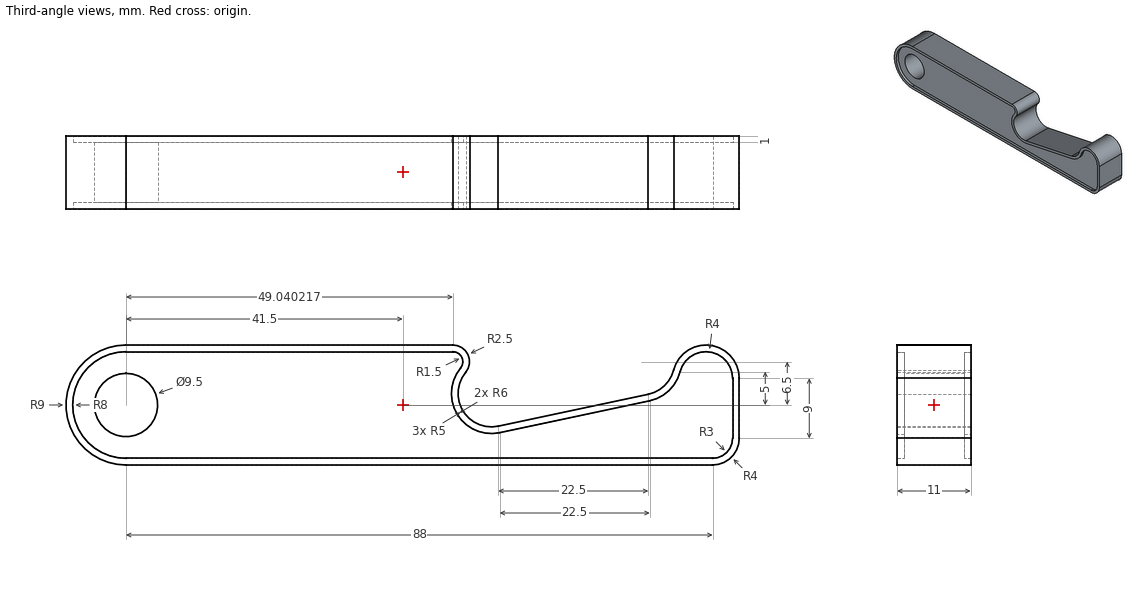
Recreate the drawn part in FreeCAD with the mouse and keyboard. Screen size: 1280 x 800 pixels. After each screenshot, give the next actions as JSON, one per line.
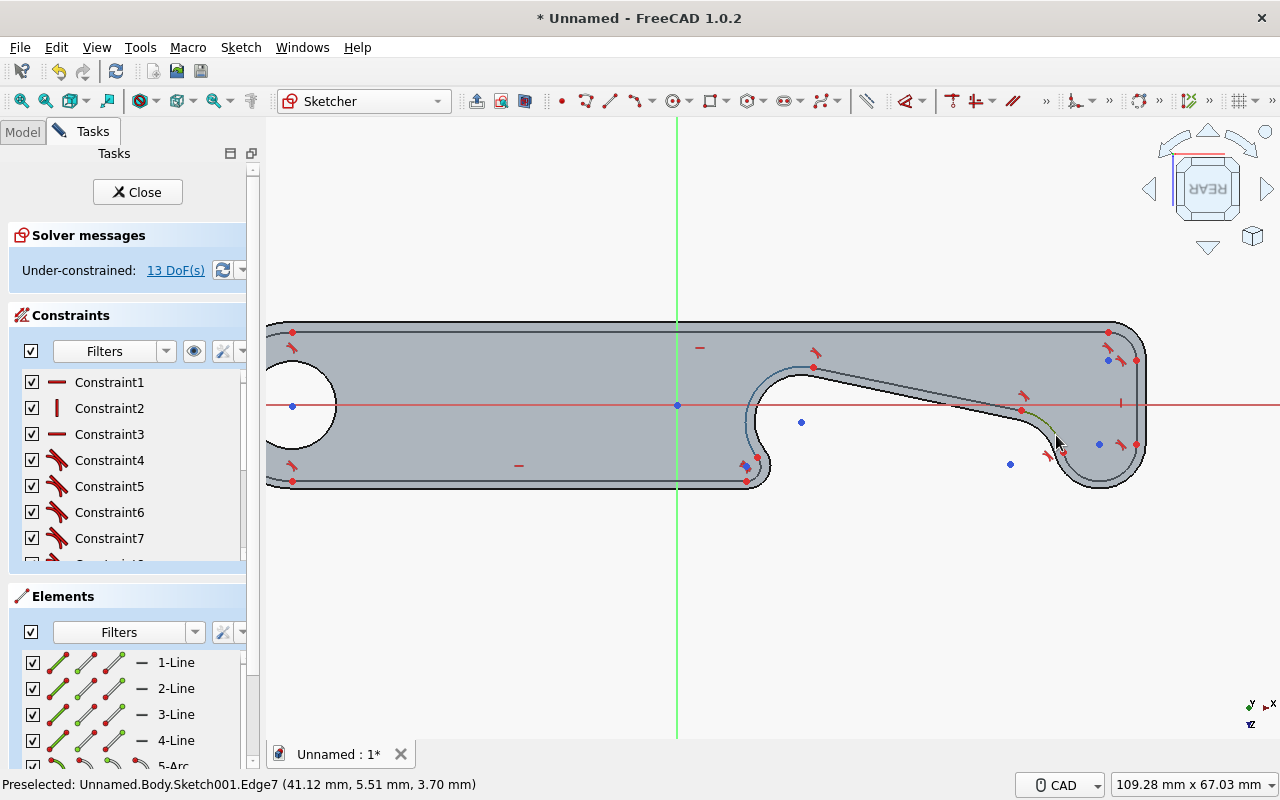
{"action": "key", "text": "e"}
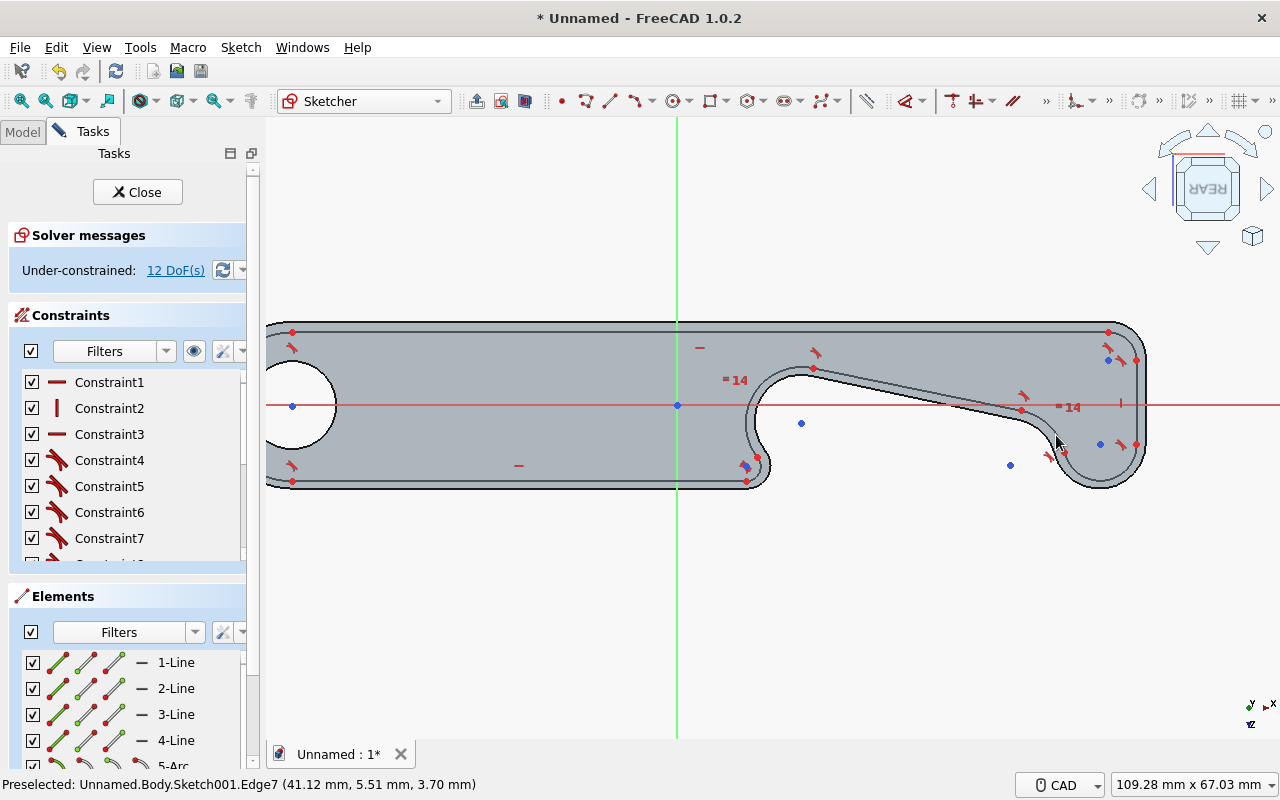
{"action": "scroll", "coordinate": [760, 474], "scroll_direction": "down", "scroll_amount": 2}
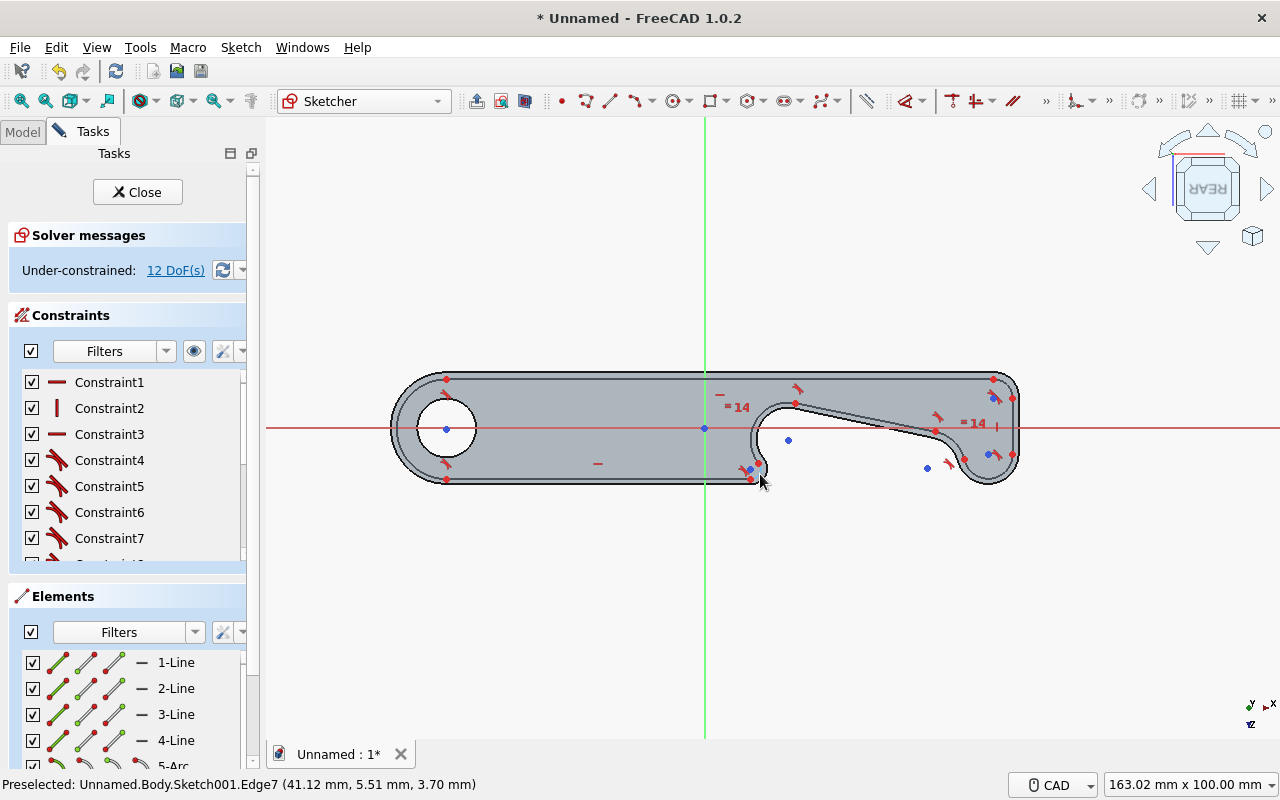
{"action": "left_click", "coordinate": [447, 429]}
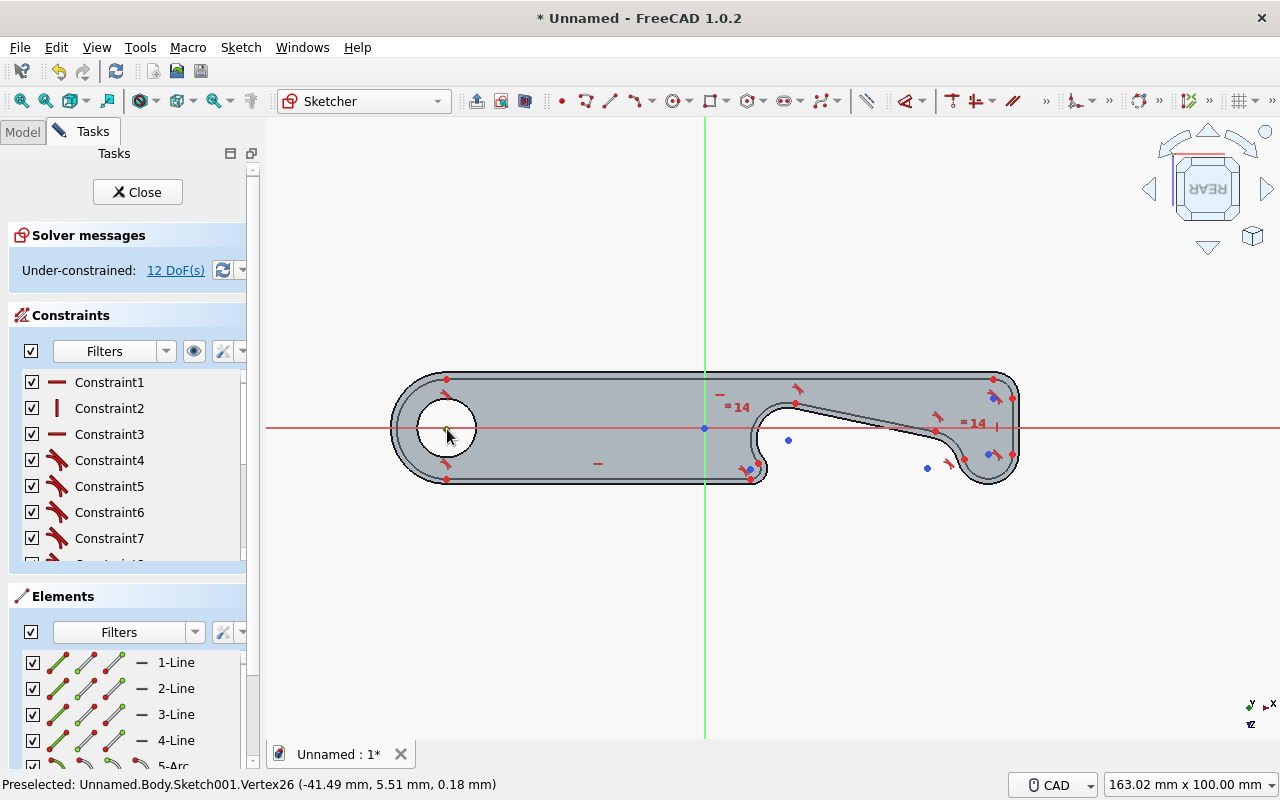
{"action": "left_click", "coordinate": [353, 428]}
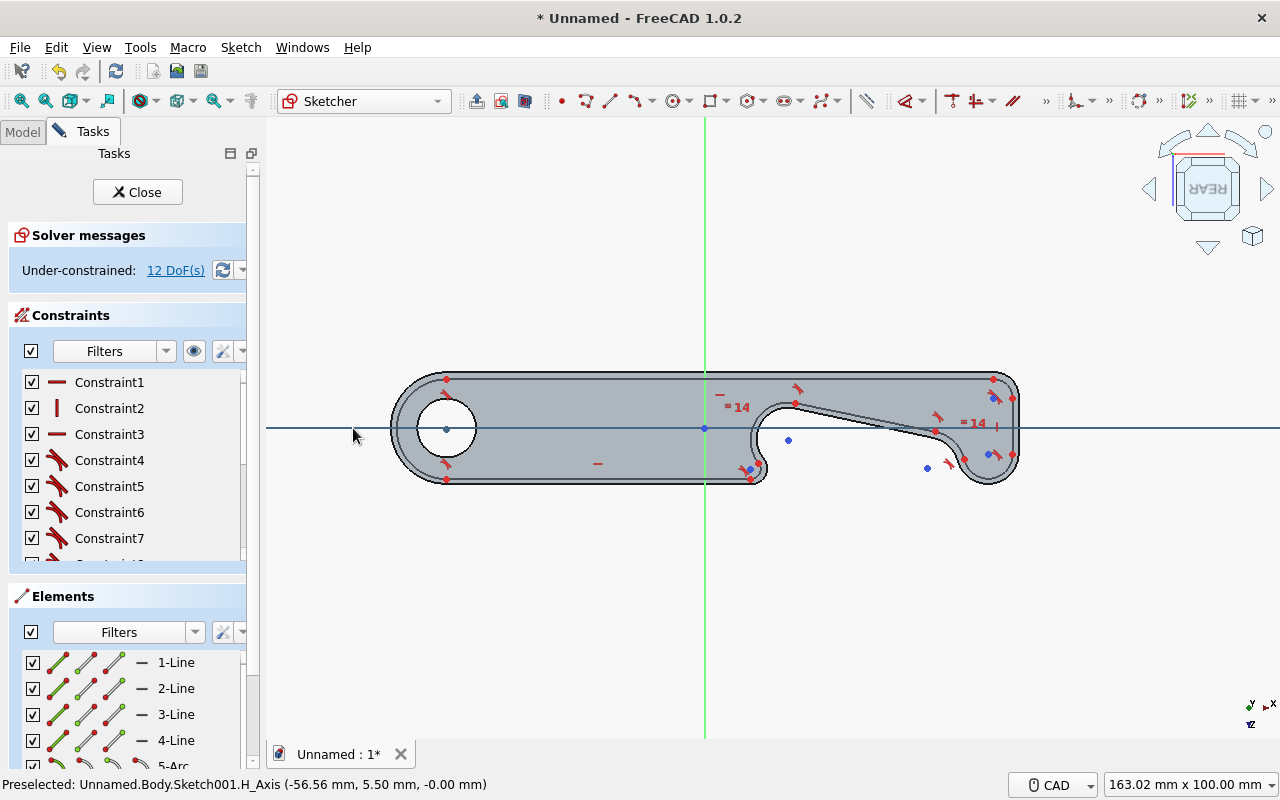
{"action": "left_click", "coordinate": [952, 102]}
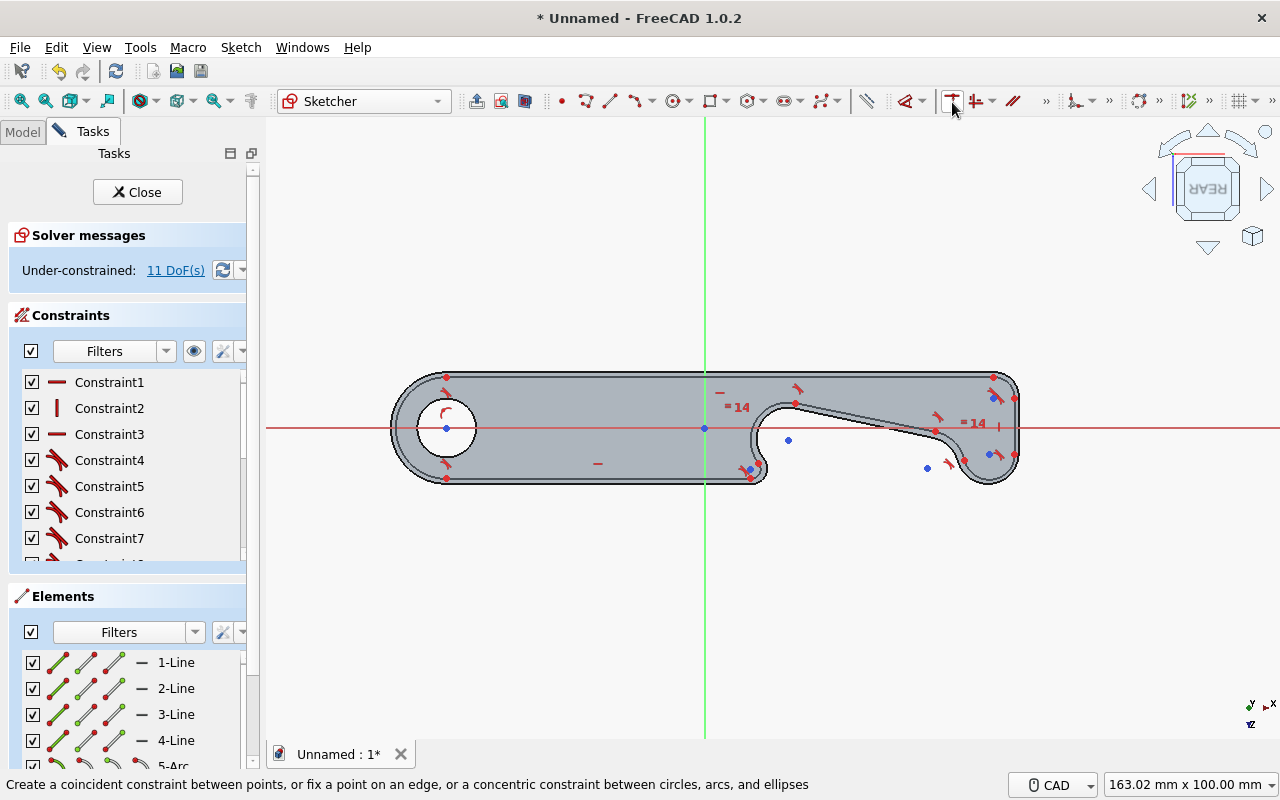
{"action": "left_click", "coordinate": [906, 102]}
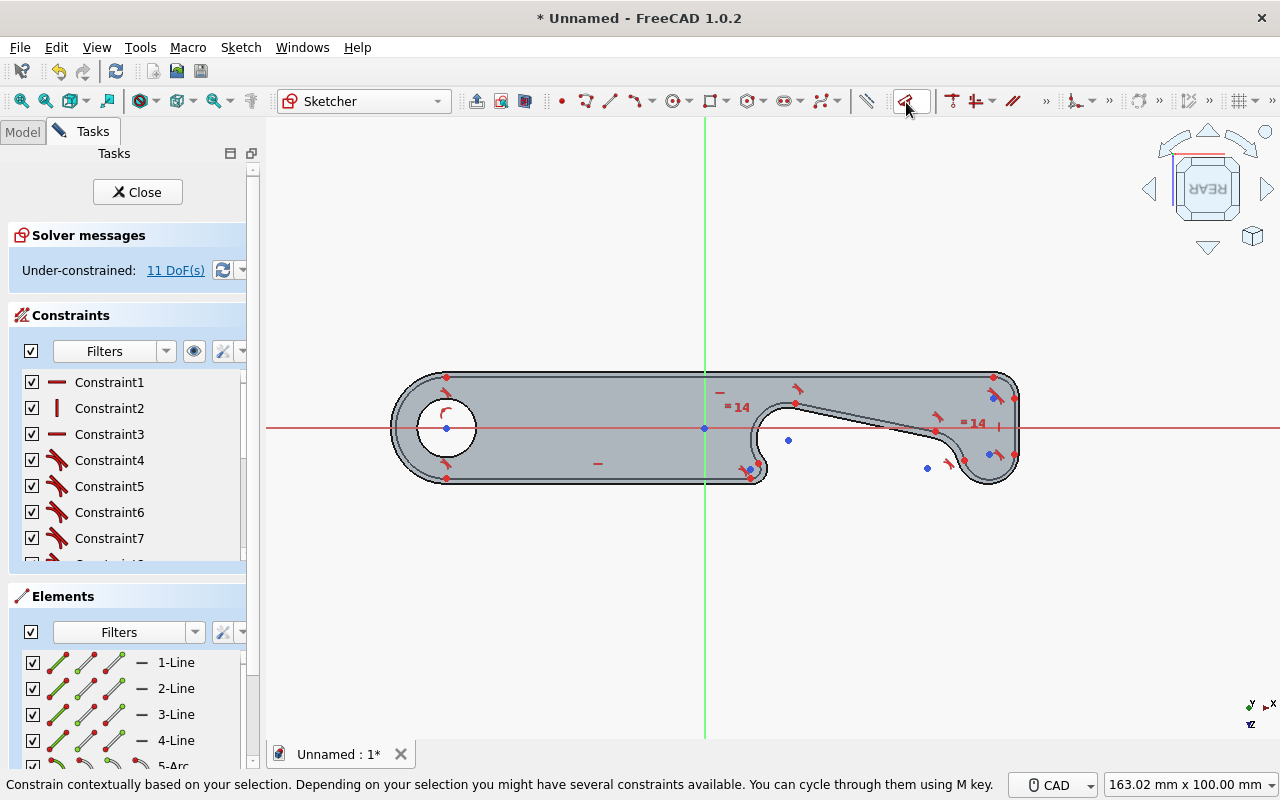
{"action": "scroll", "coordinate": [760, 473], "scroll_direction": "up", "scroll_amount": 8}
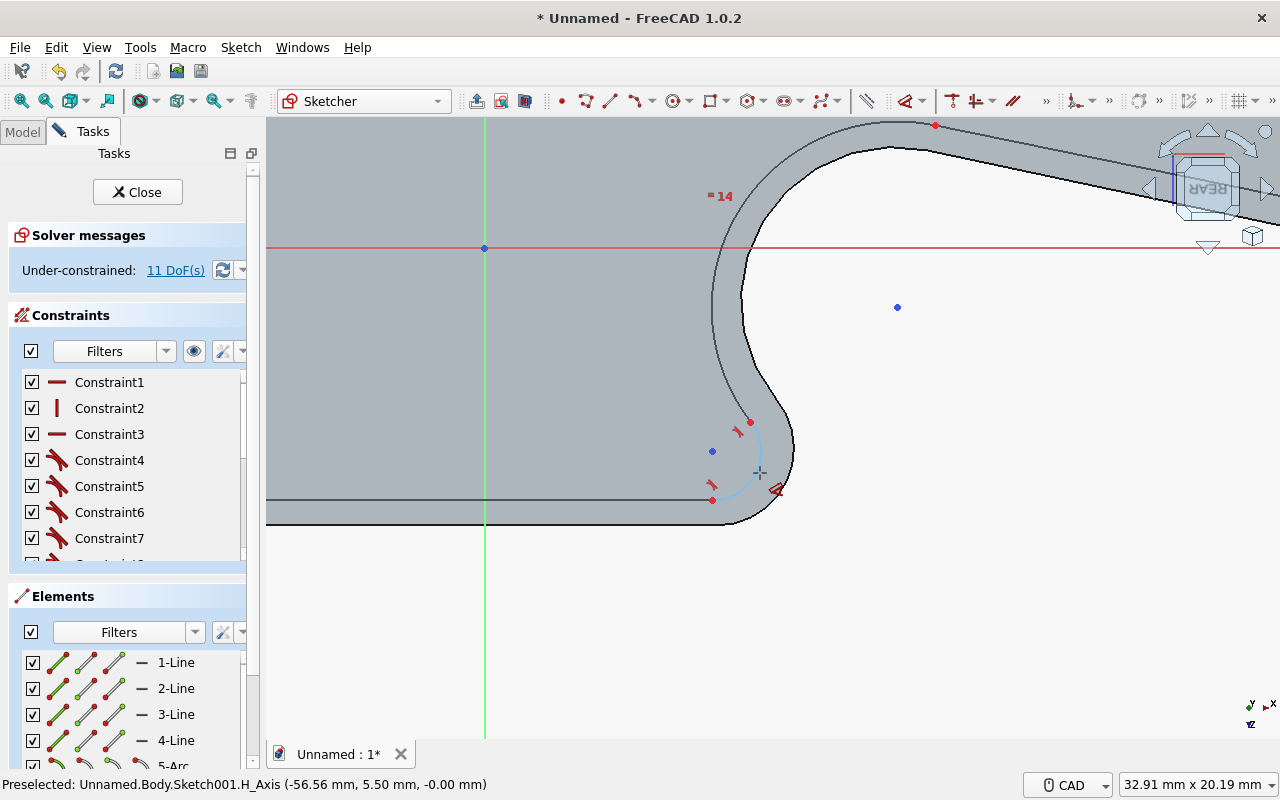
{"action": "left_click", "coordinate": [756, 473]}
{"action": "left_click", "coordinate": [785, 487]}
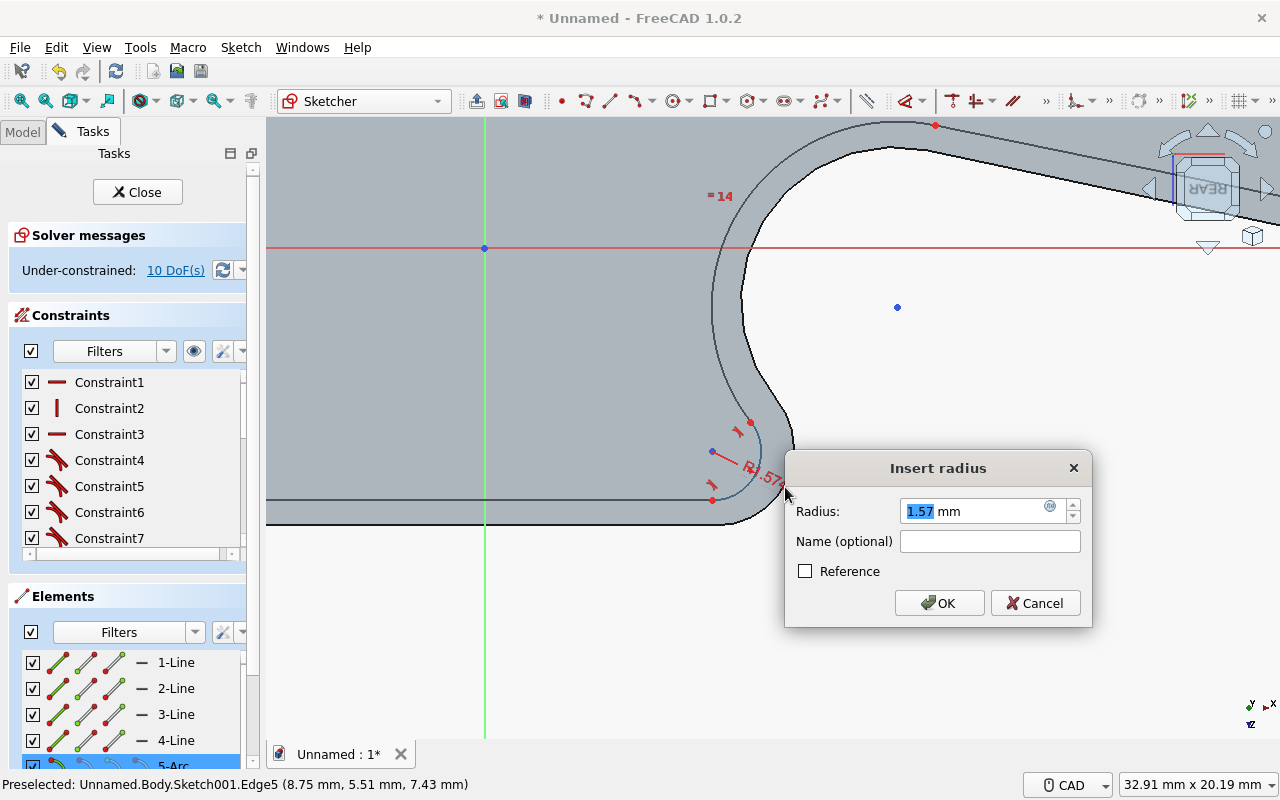
{"action": "type", "text": "1.5"}
{"action": "key", "text": "Return"}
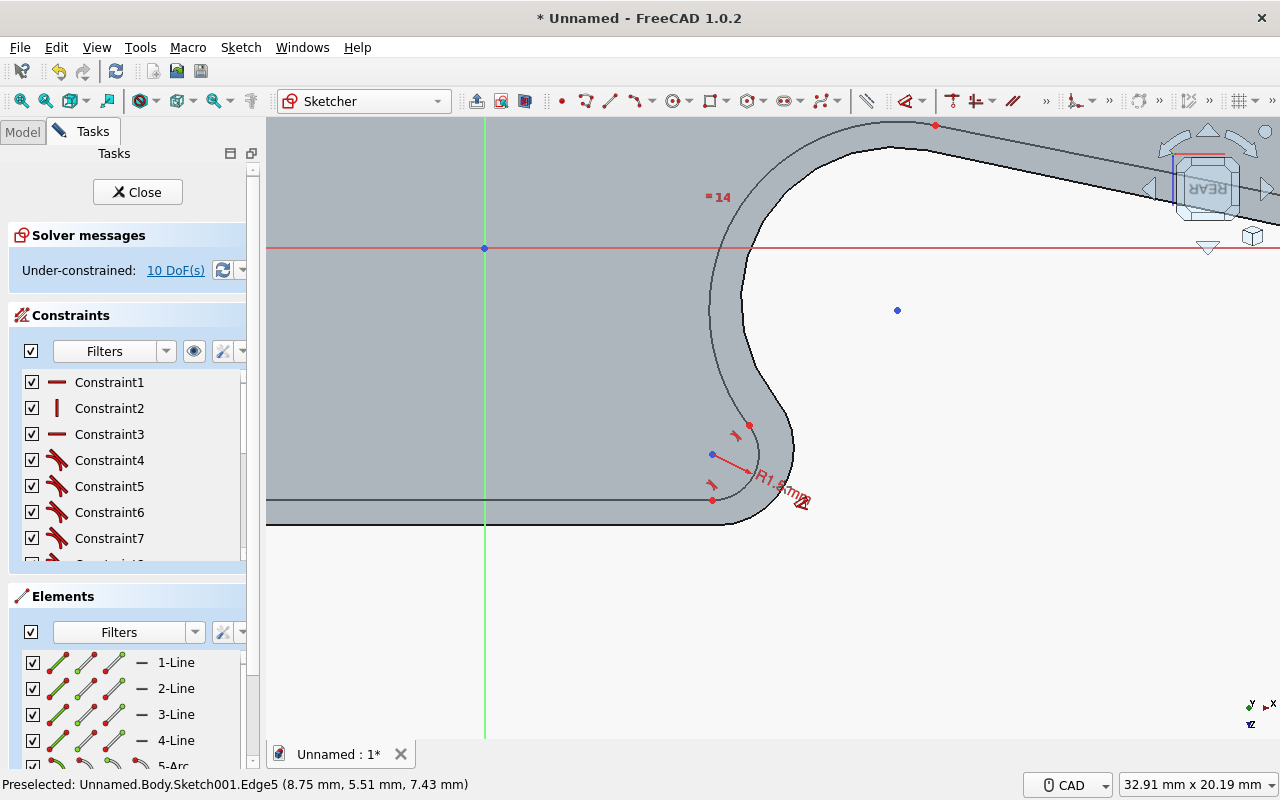
{"action": "scroll", "coordinate": [760, 474], "scroll_direction": "down", "scroll_amount": 8}